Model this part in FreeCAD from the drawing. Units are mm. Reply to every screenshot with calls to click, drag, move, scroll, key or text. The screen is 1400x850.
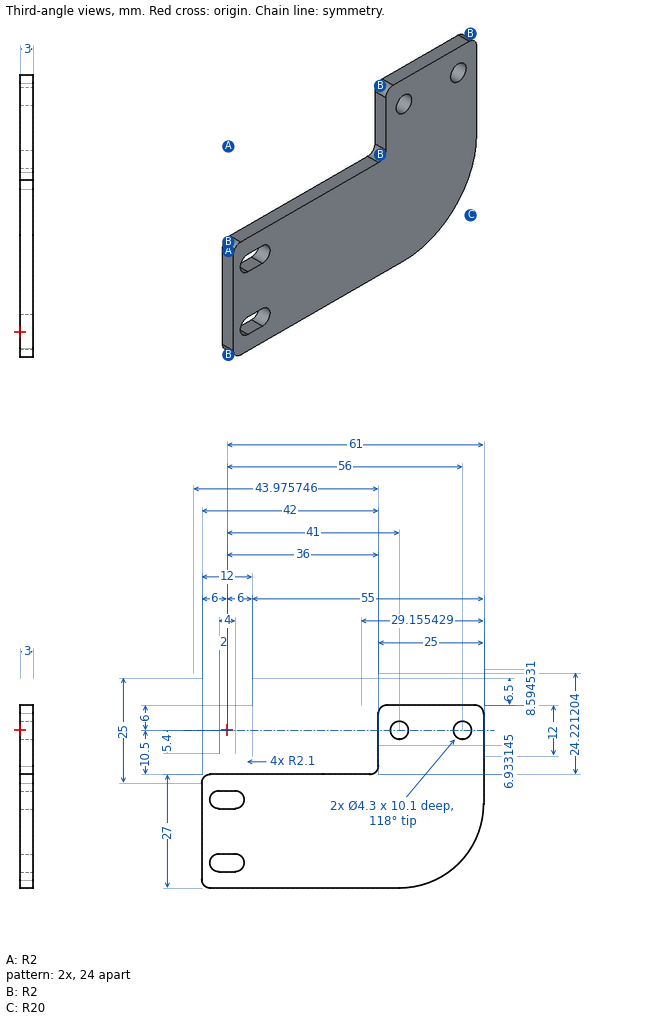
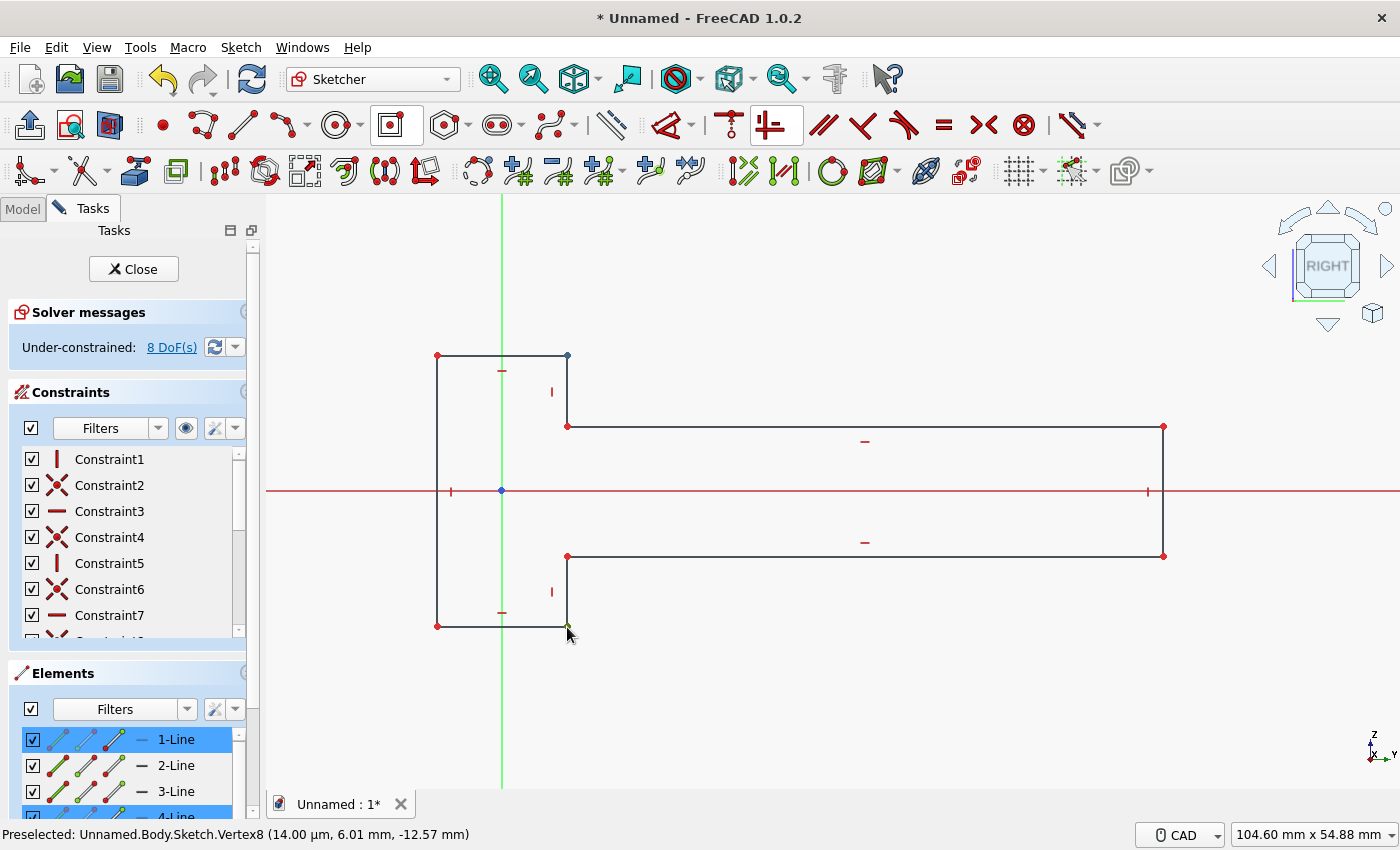
click(361, 491)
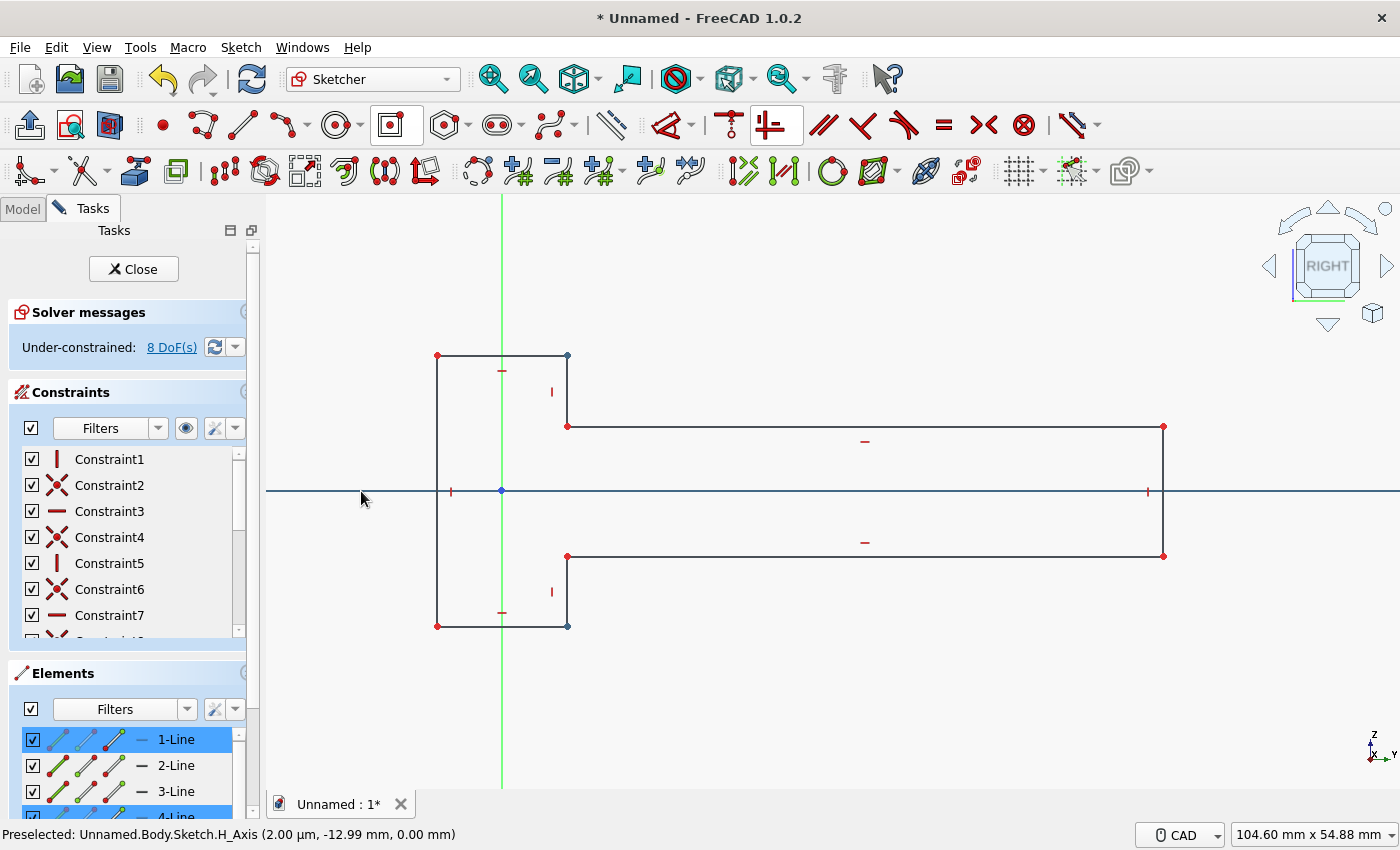
click(984, 126)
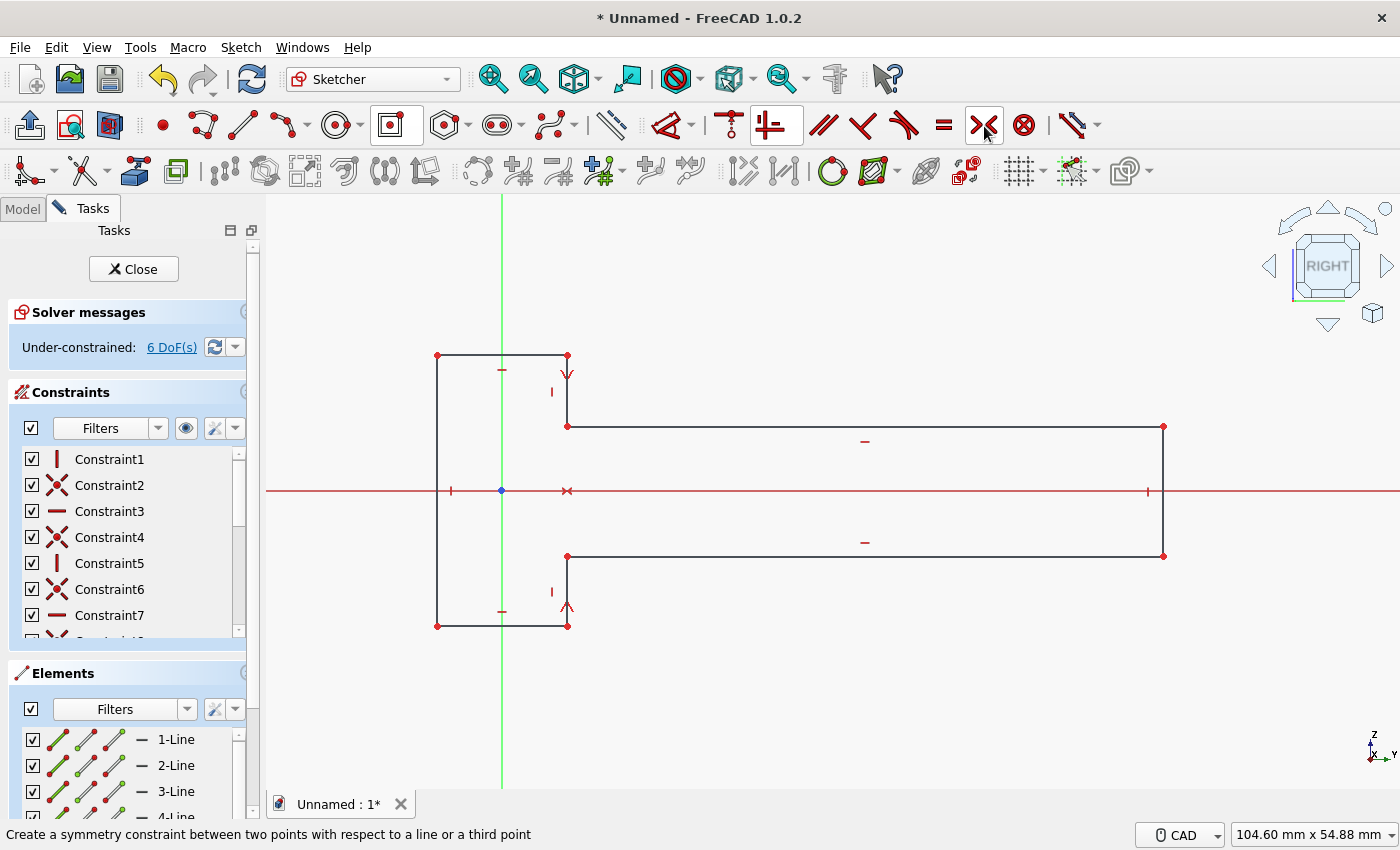
key(d)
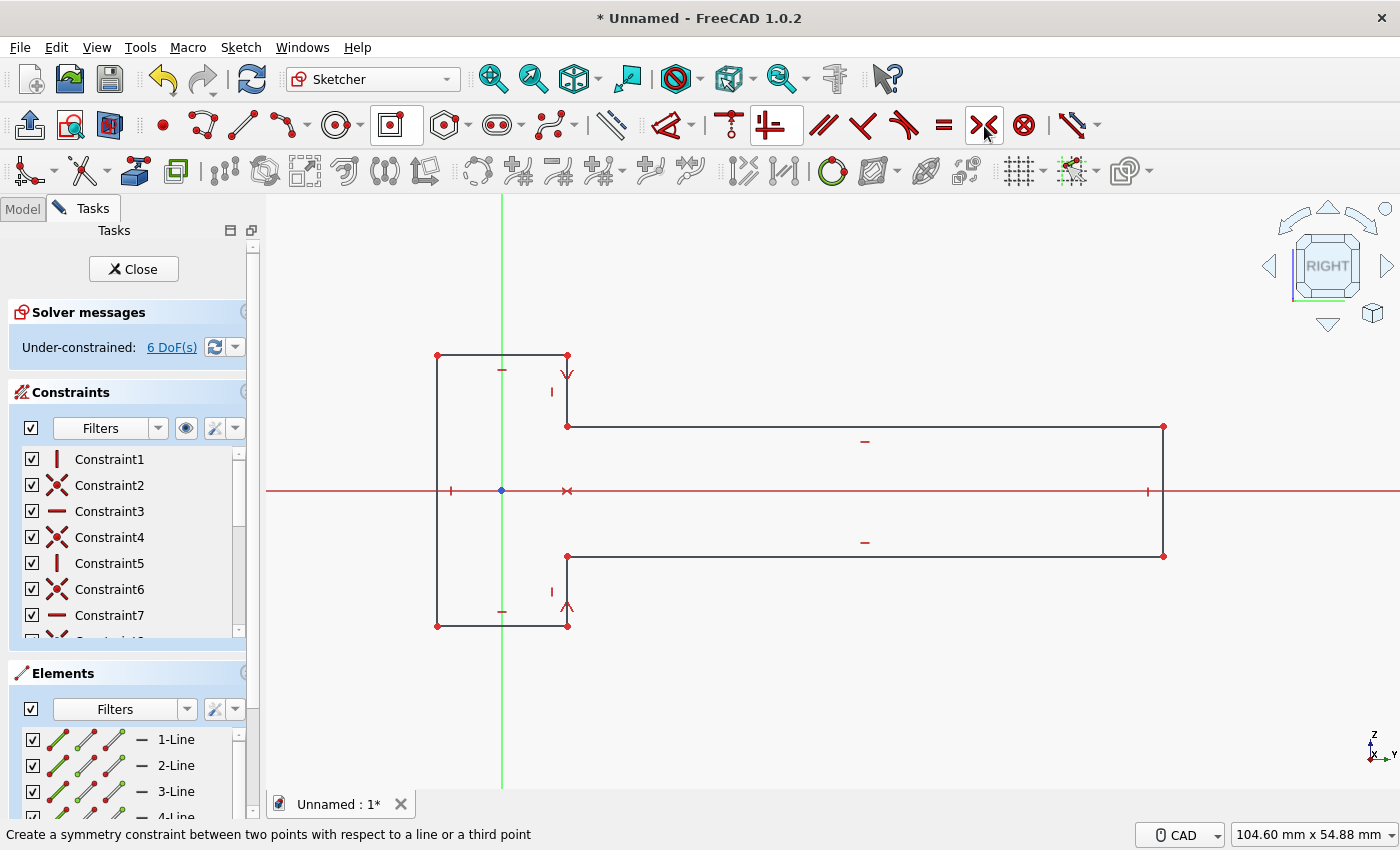
click(528, 355)
click(472, 321)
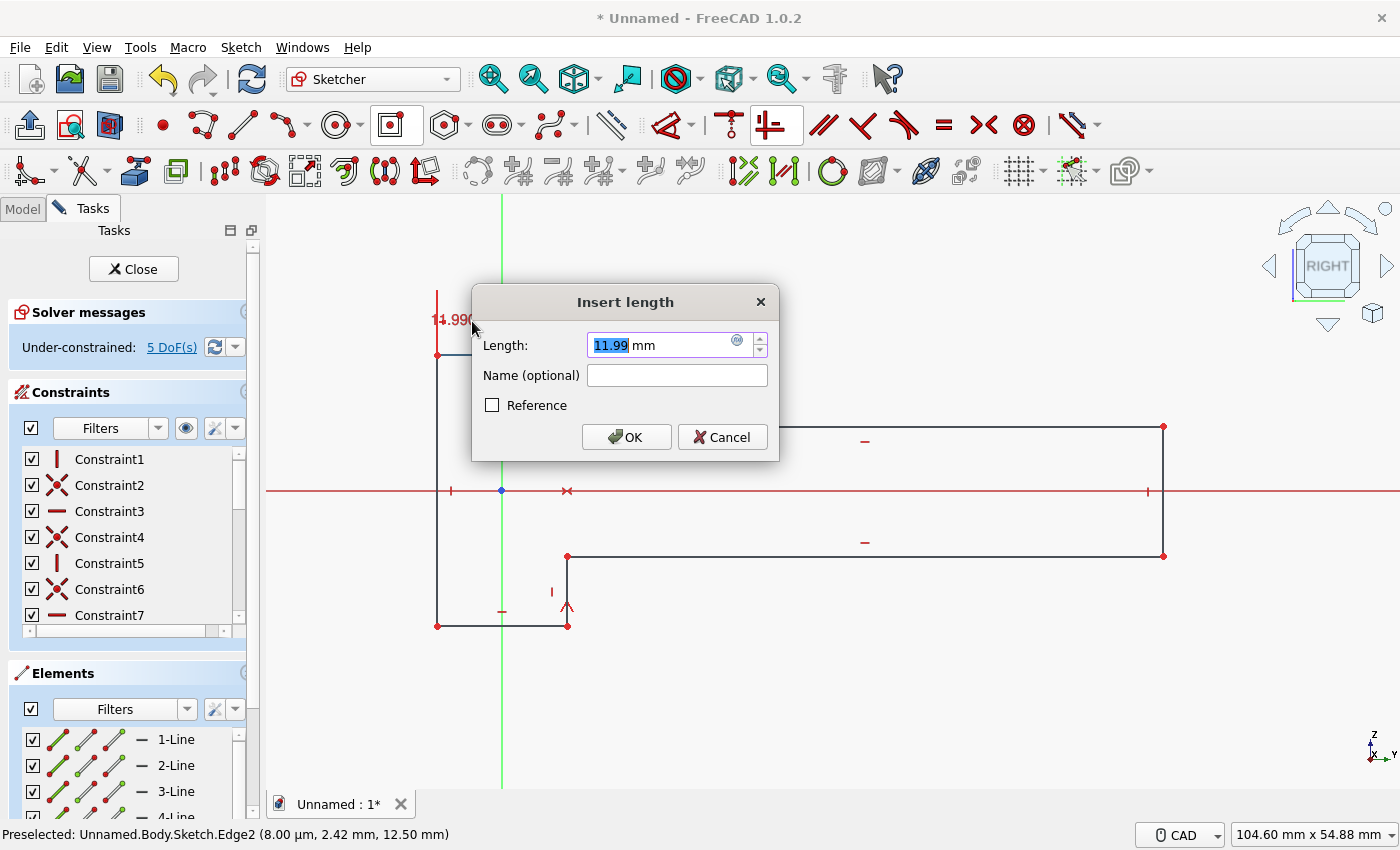
text(12)
key(Return)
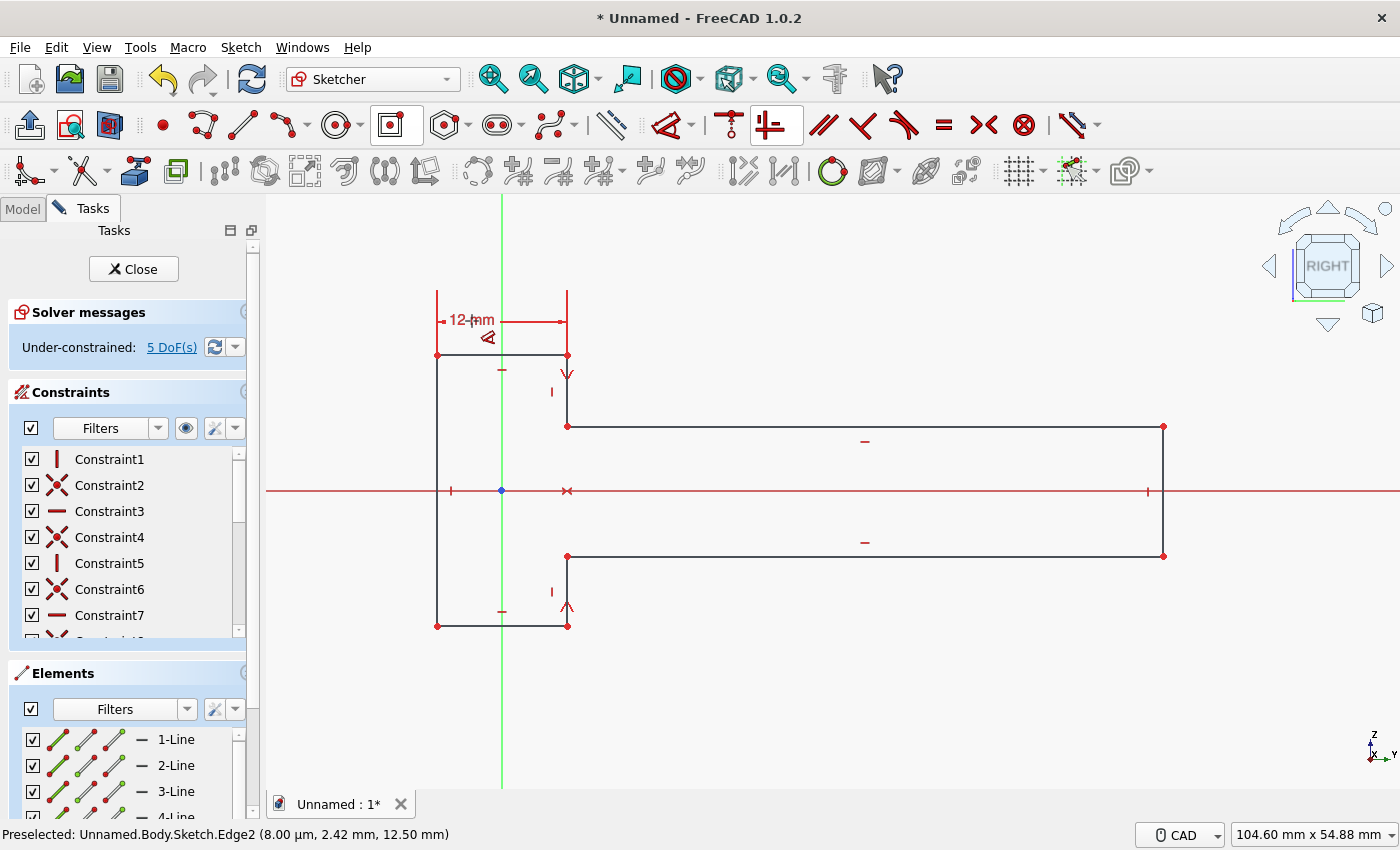
click(437, 436)
click(403, 428)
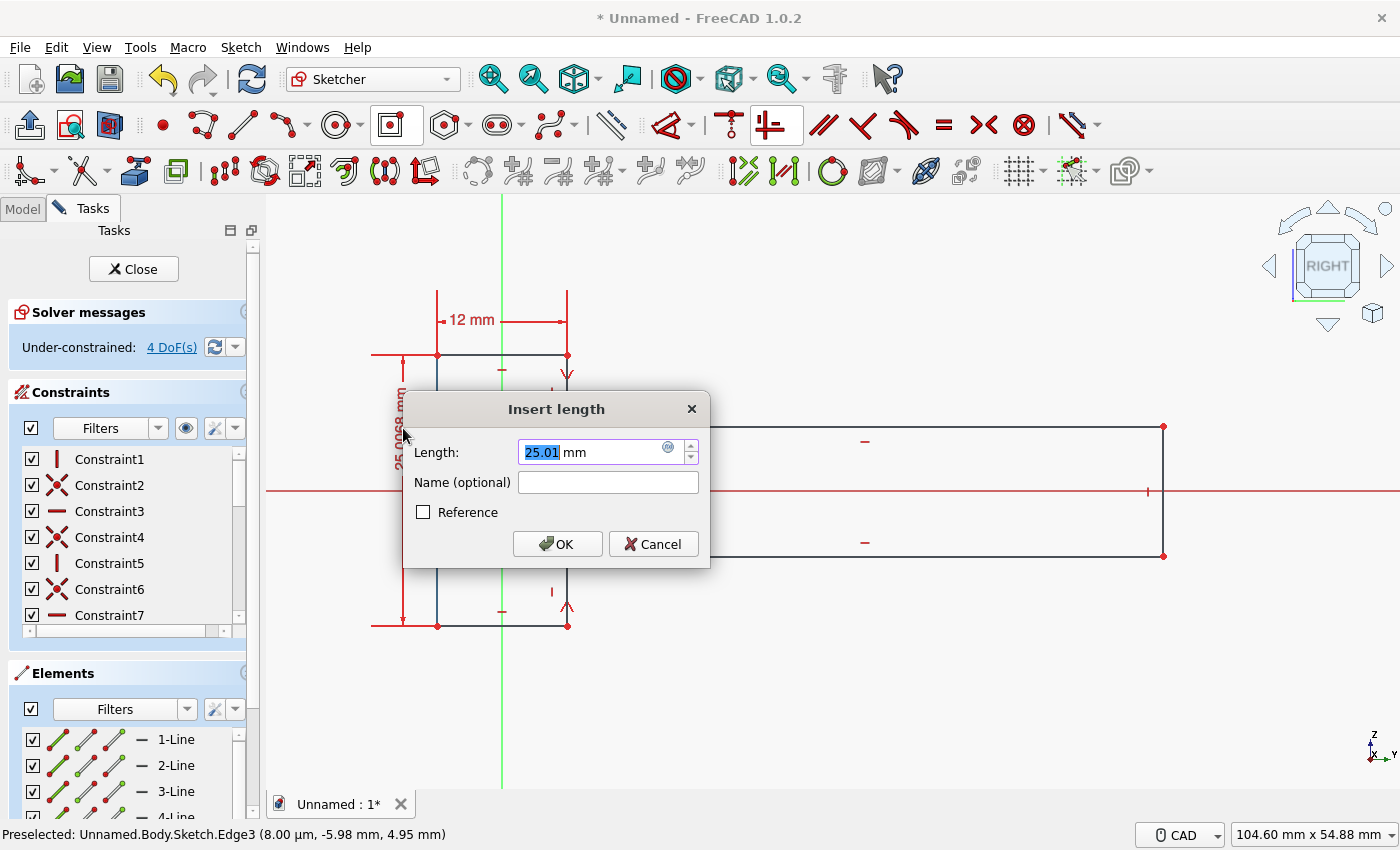
text(25)
key(Return)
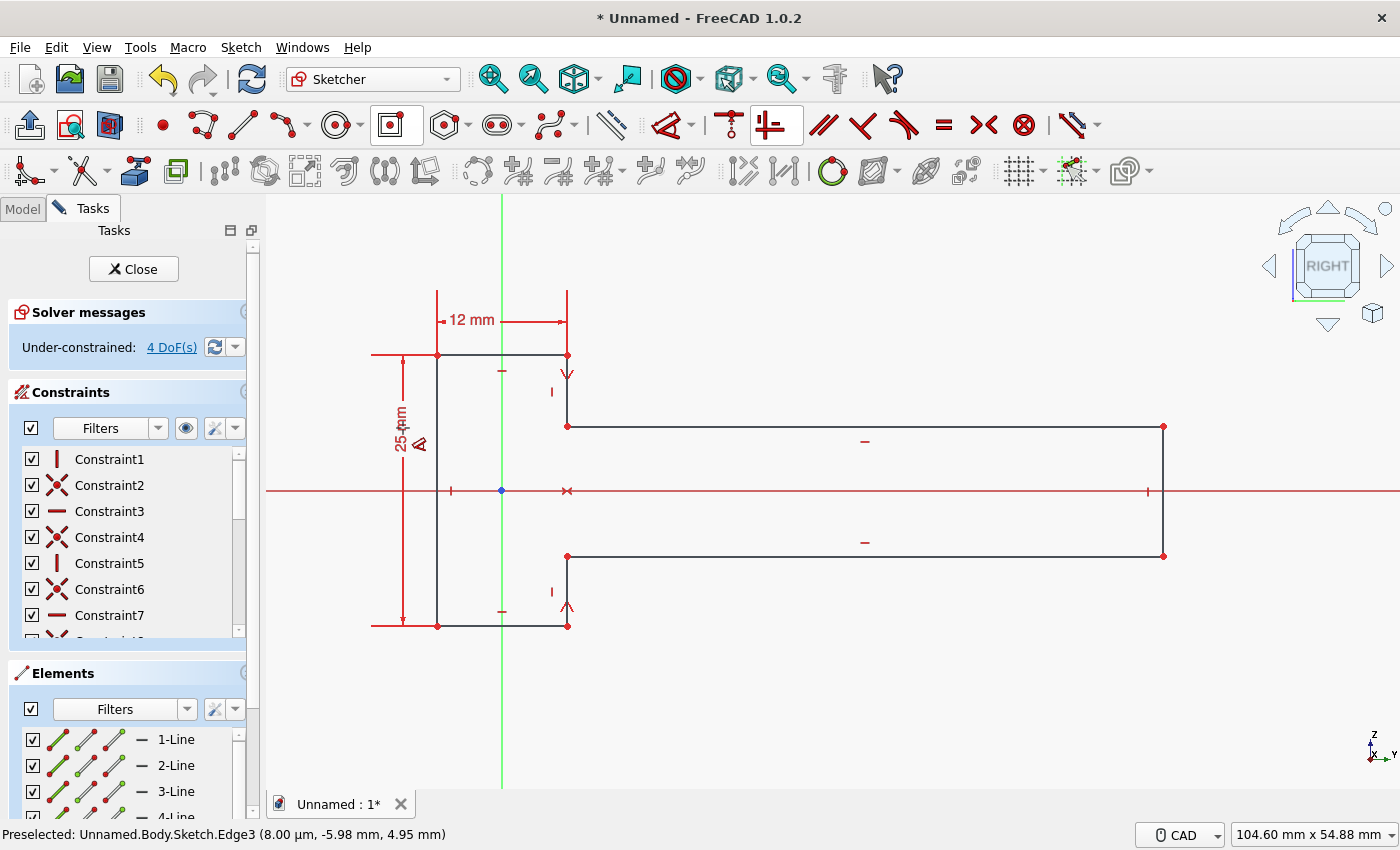
click(746, 557)
click(865, 591)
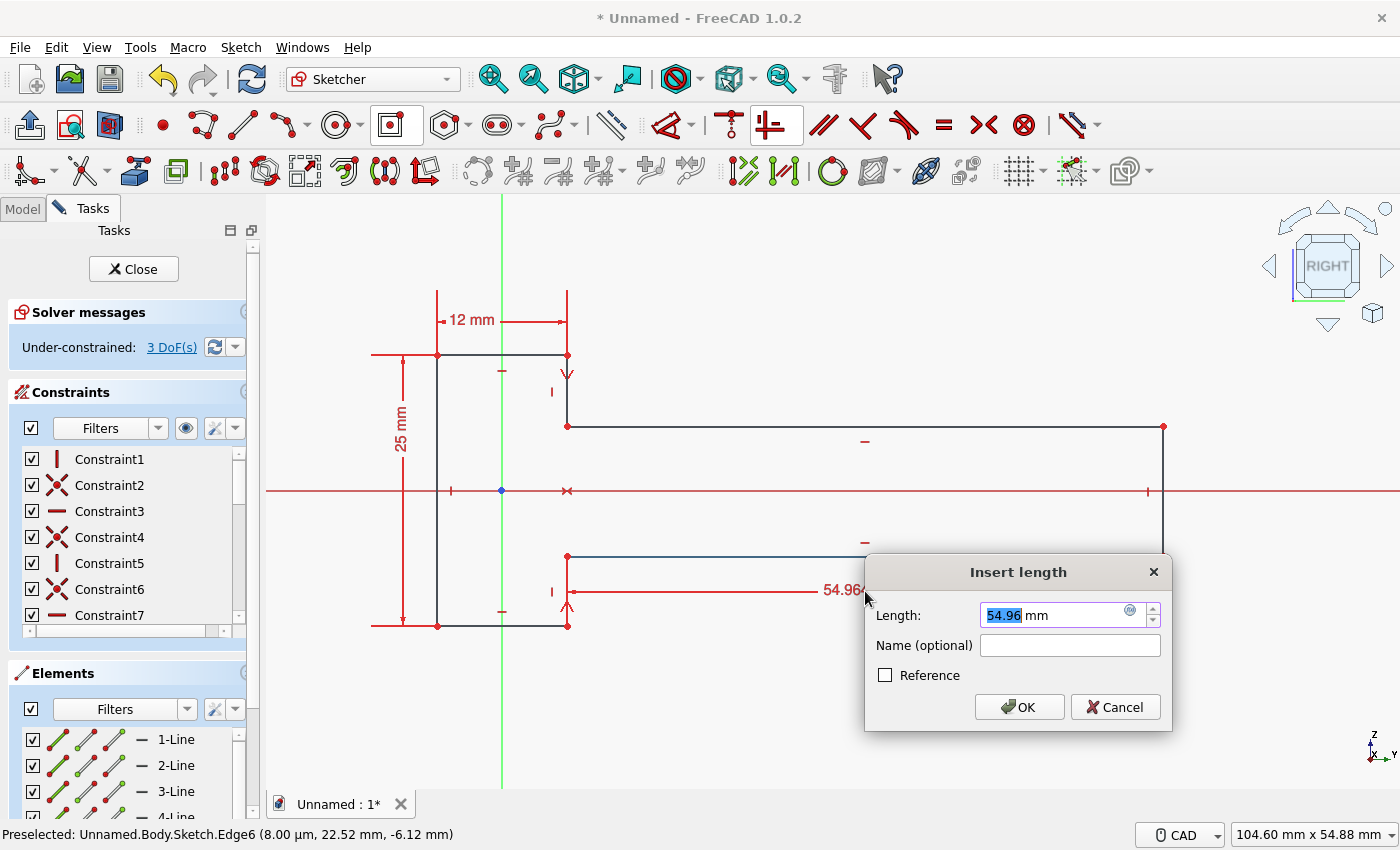
text(55)
key(Return)